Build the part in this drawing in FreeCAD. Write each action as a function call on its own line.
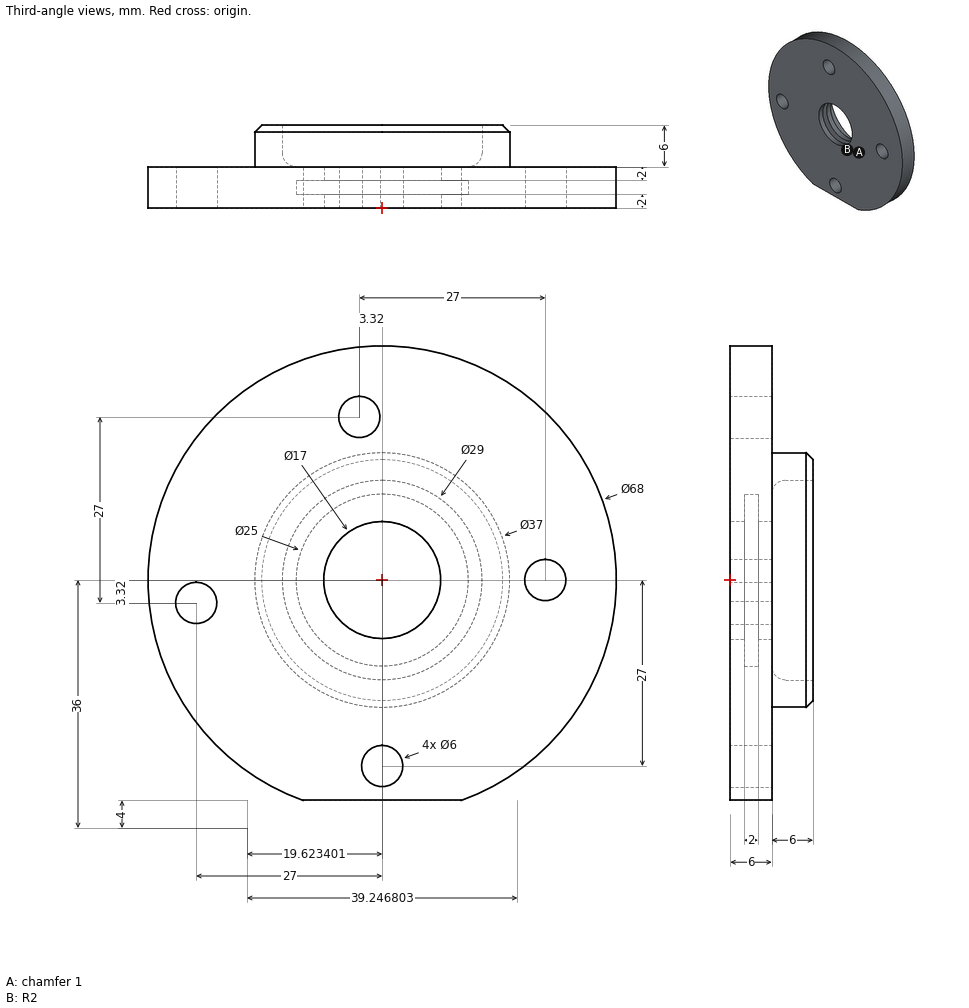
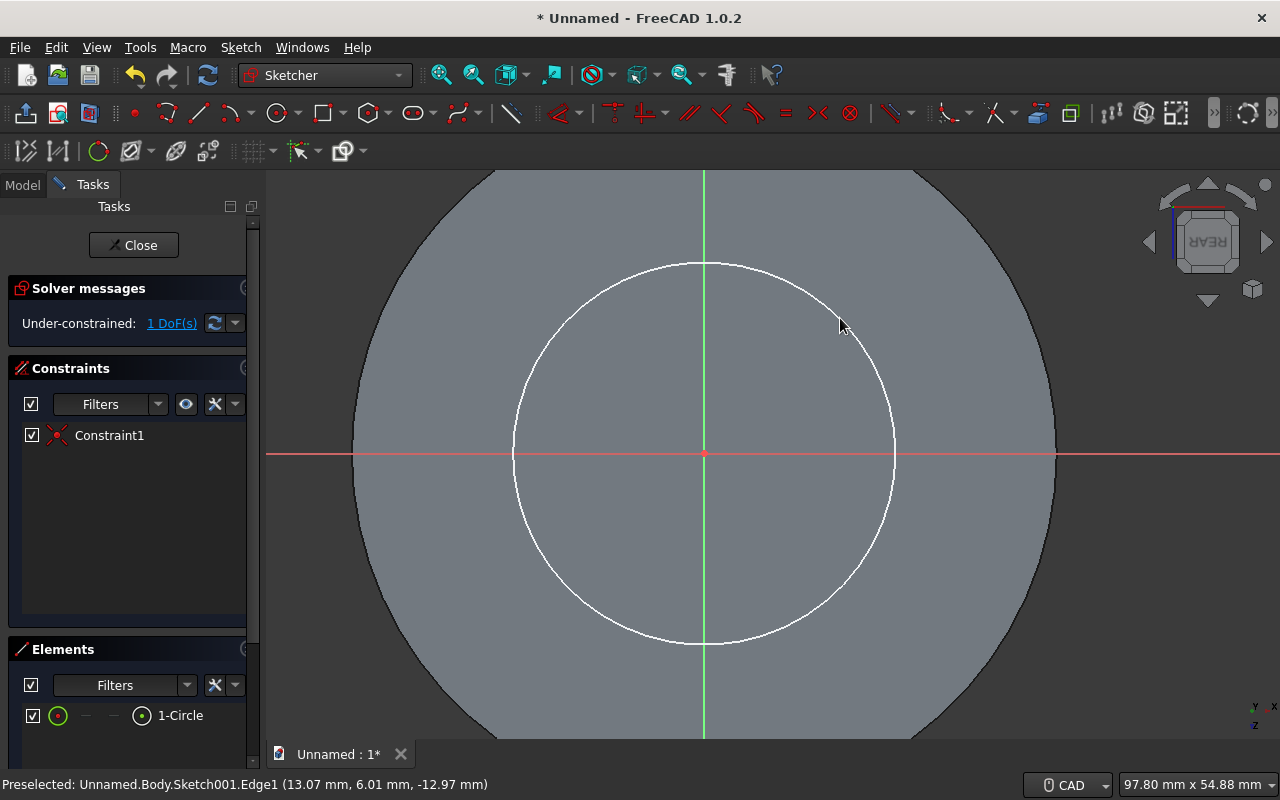
click(558, 114)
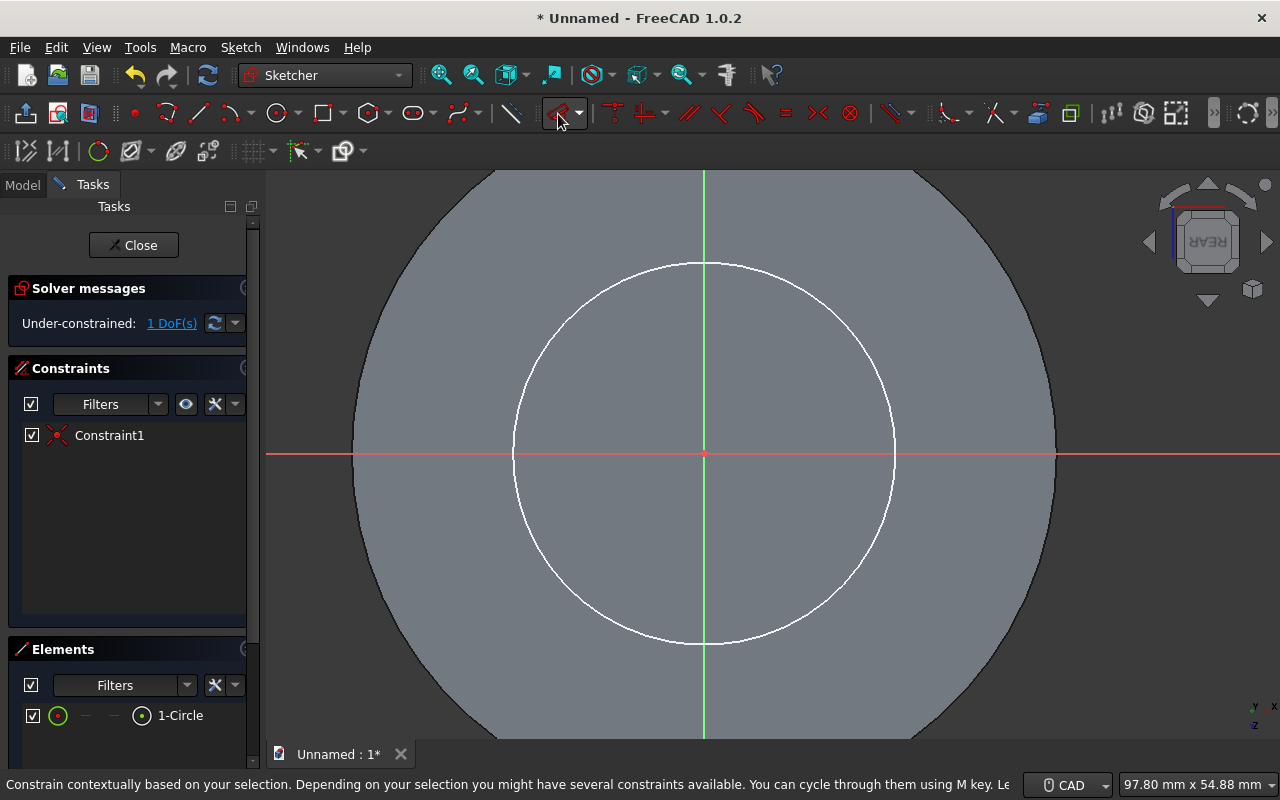
click(839, 318)
click(862, 295)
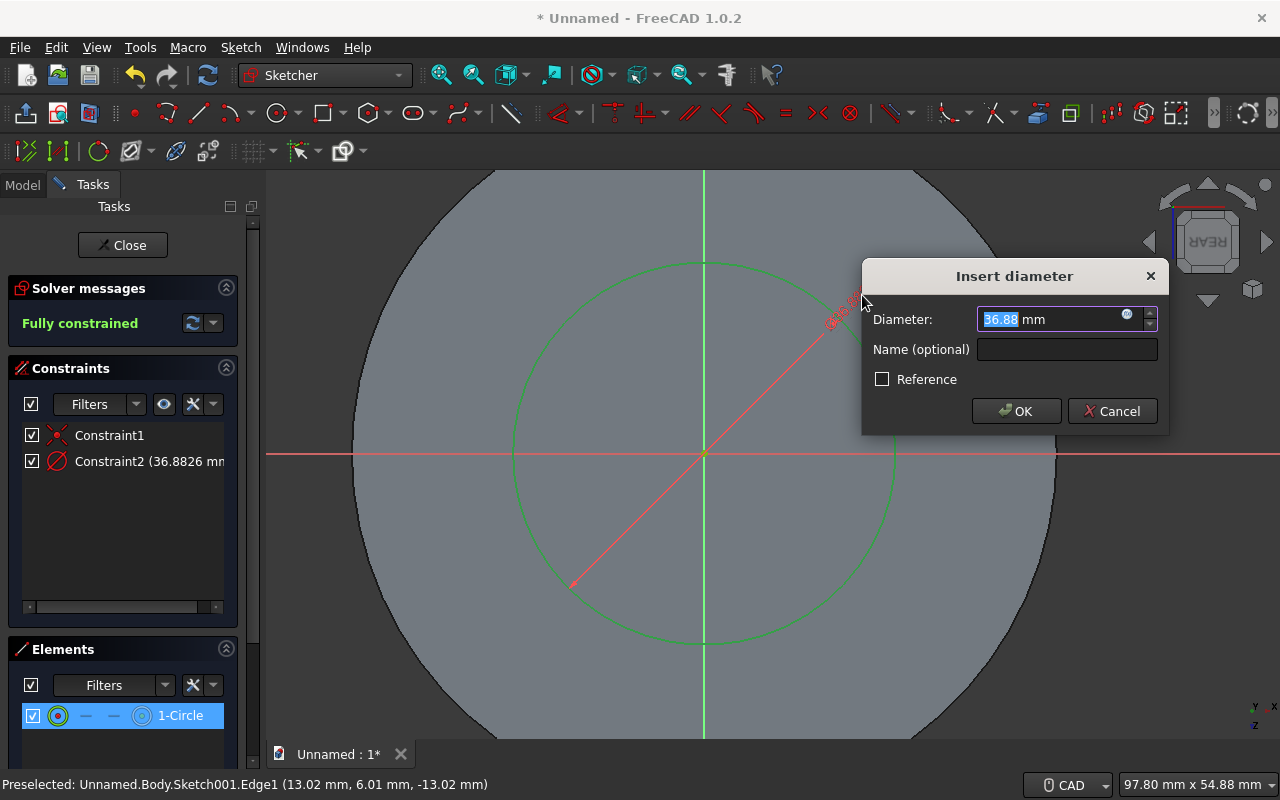
text(37)
key(Return)
key(Escape)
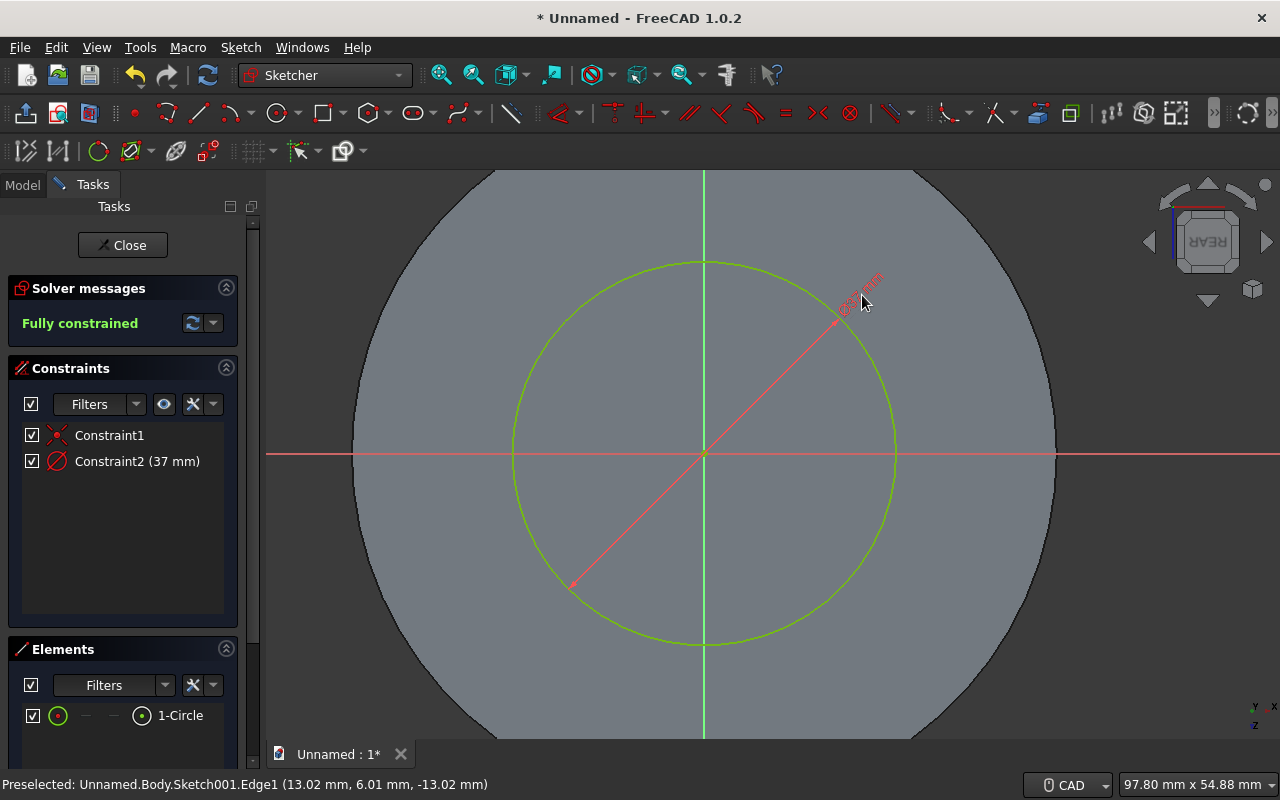
click(123, 245)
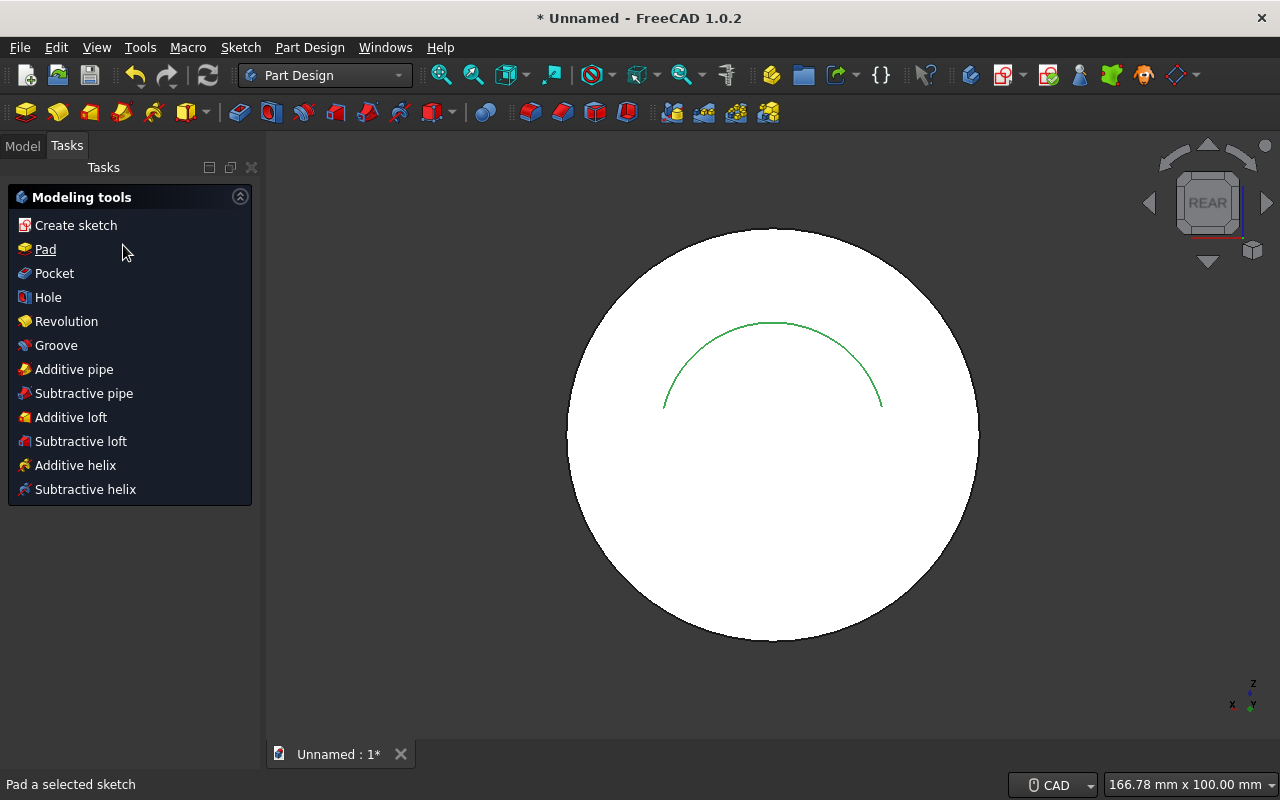
click(26, 112)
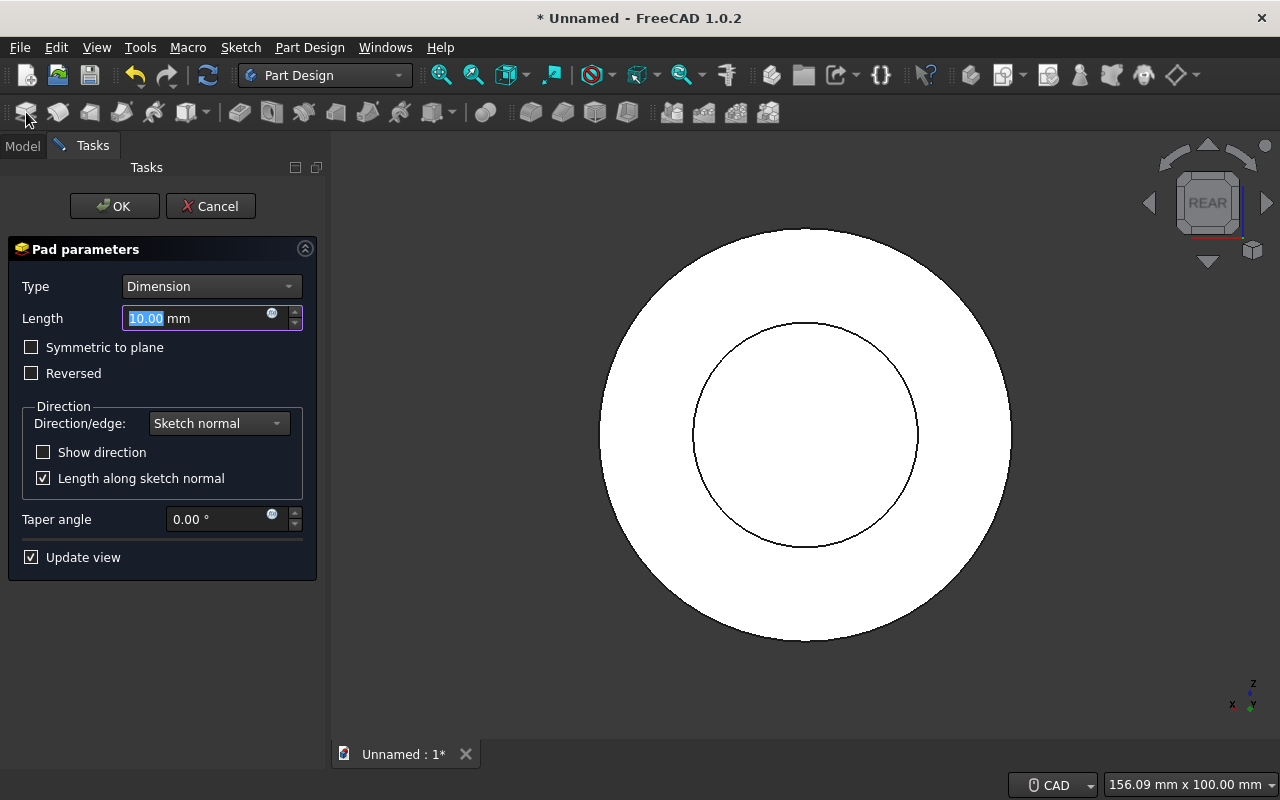
text(6)
key(Tab)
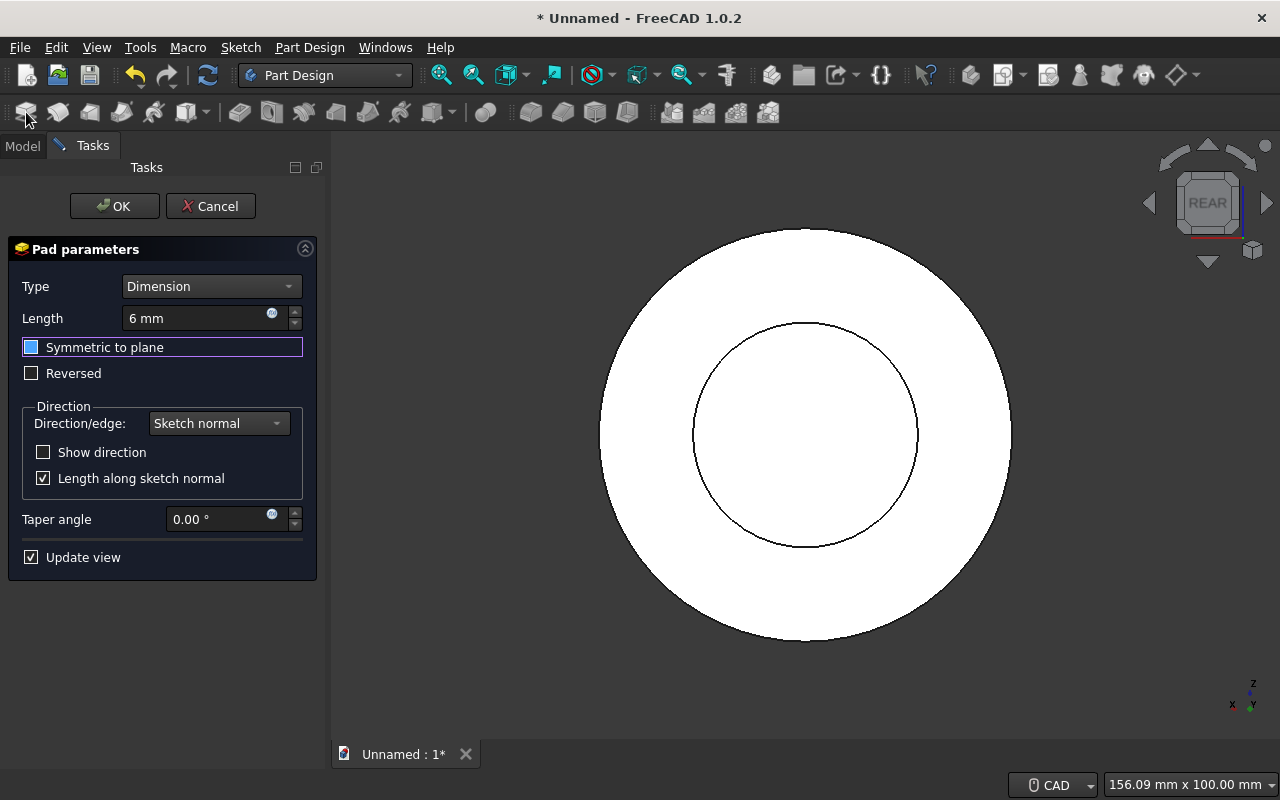
click(115, 206)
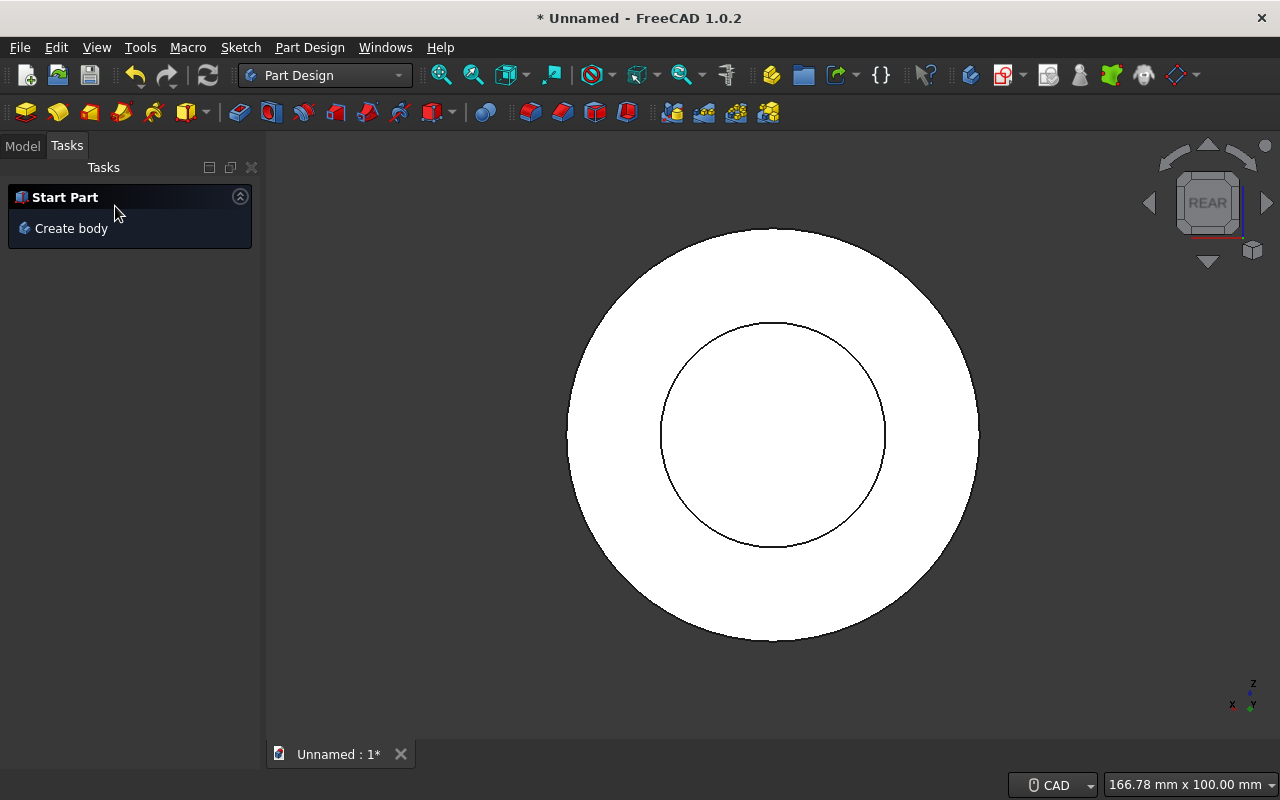
click(773, 434)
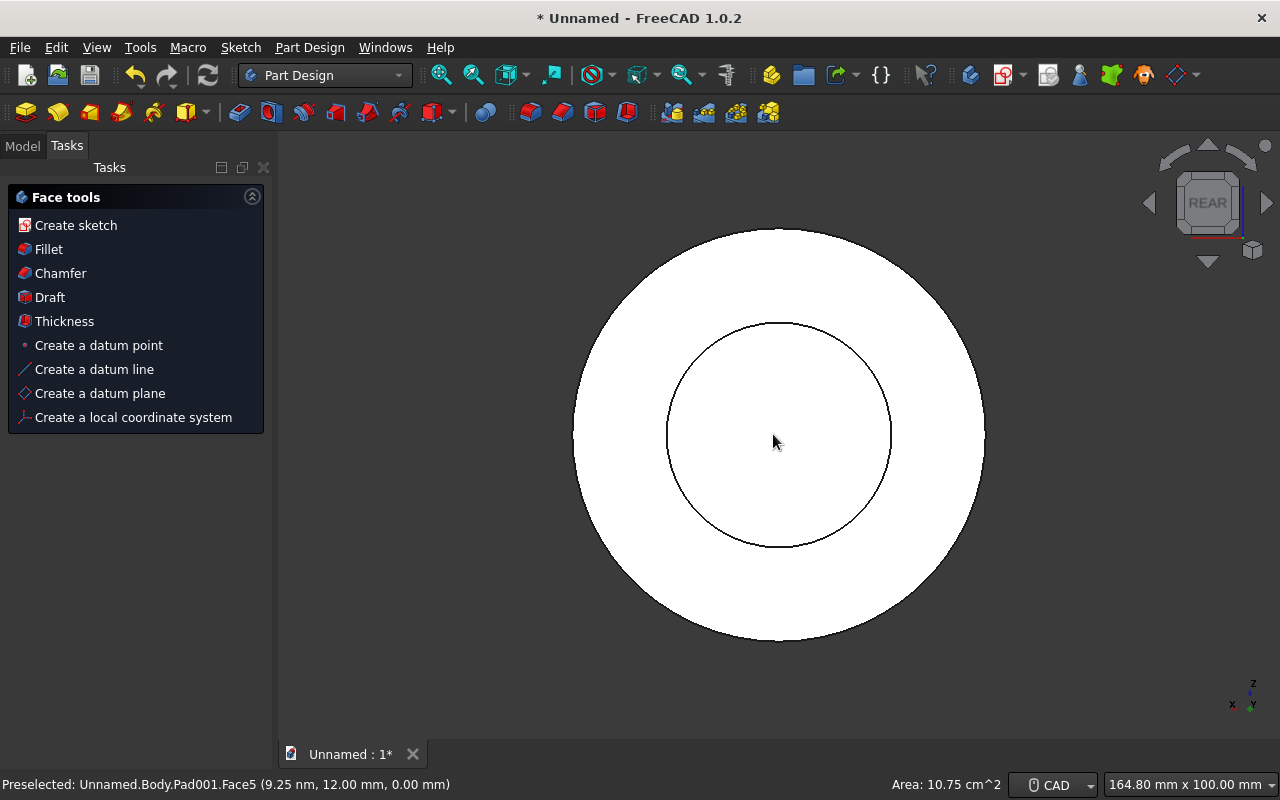
click(1004, 76)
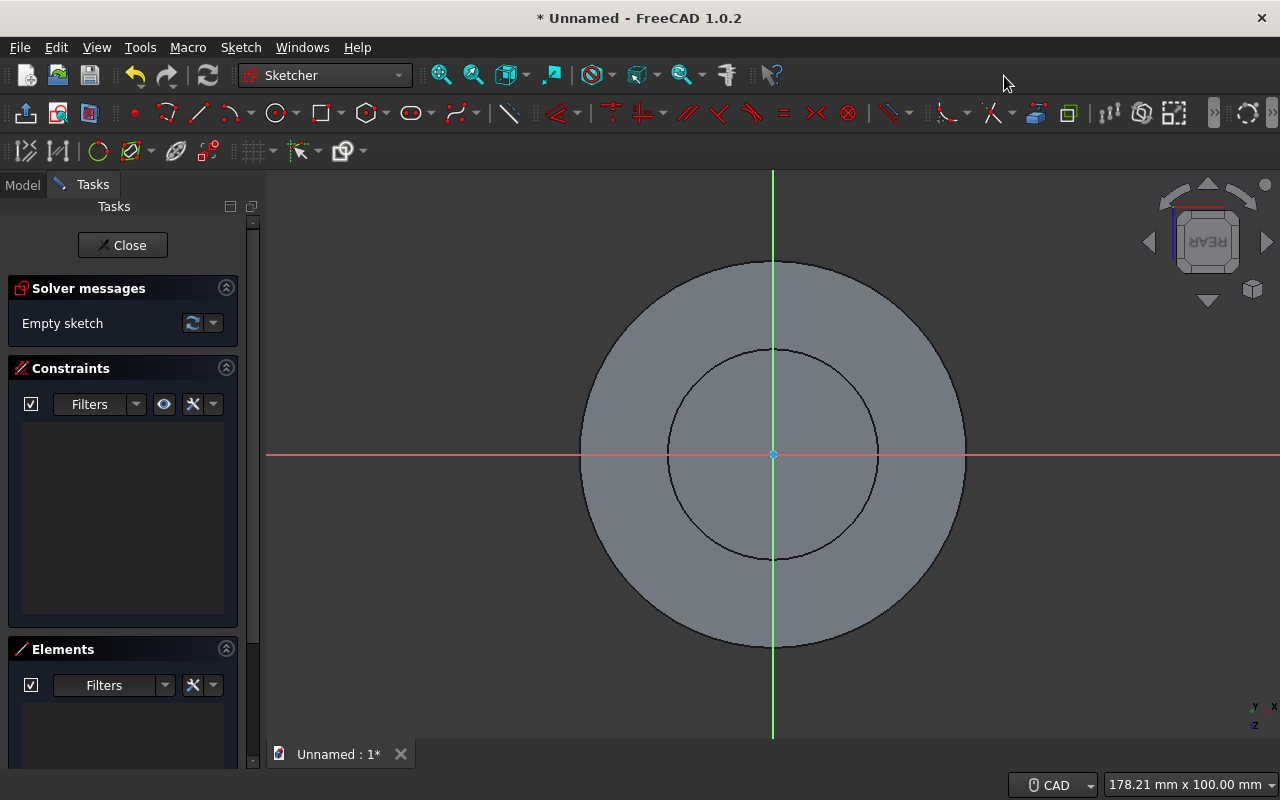
scroll(829, 454, up, 4)